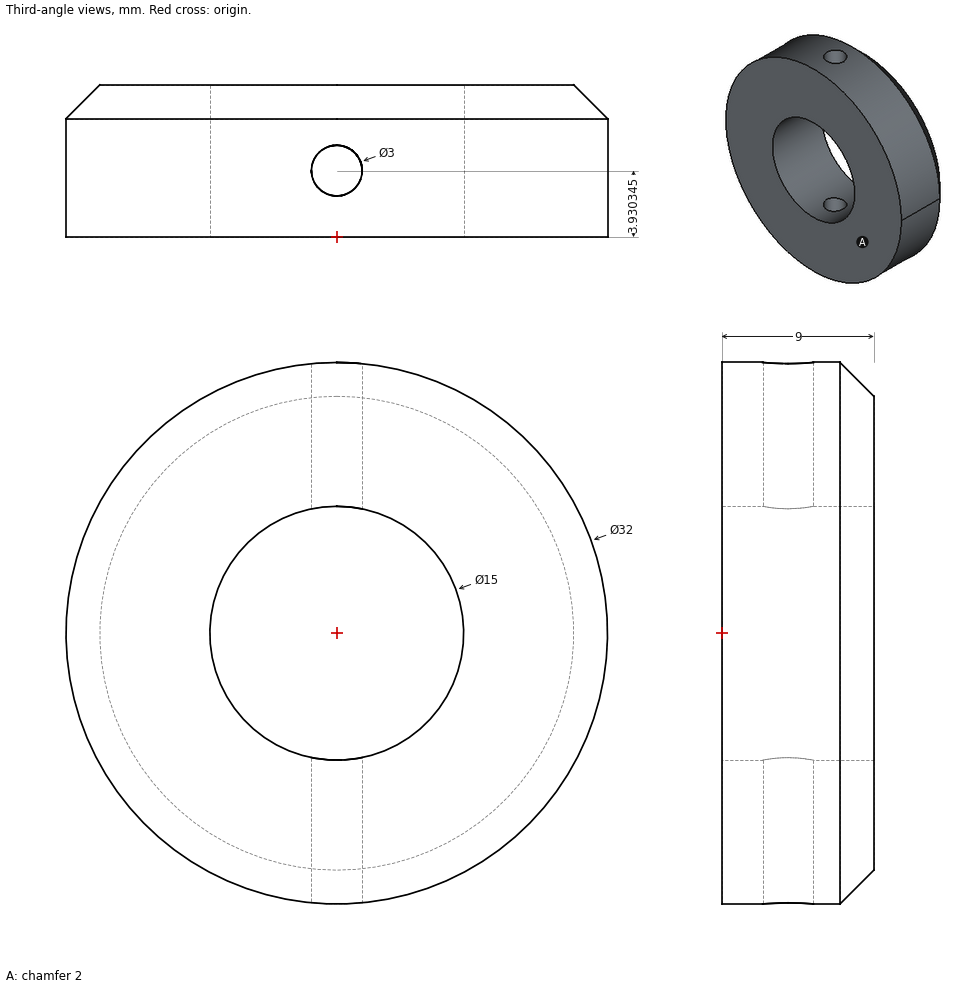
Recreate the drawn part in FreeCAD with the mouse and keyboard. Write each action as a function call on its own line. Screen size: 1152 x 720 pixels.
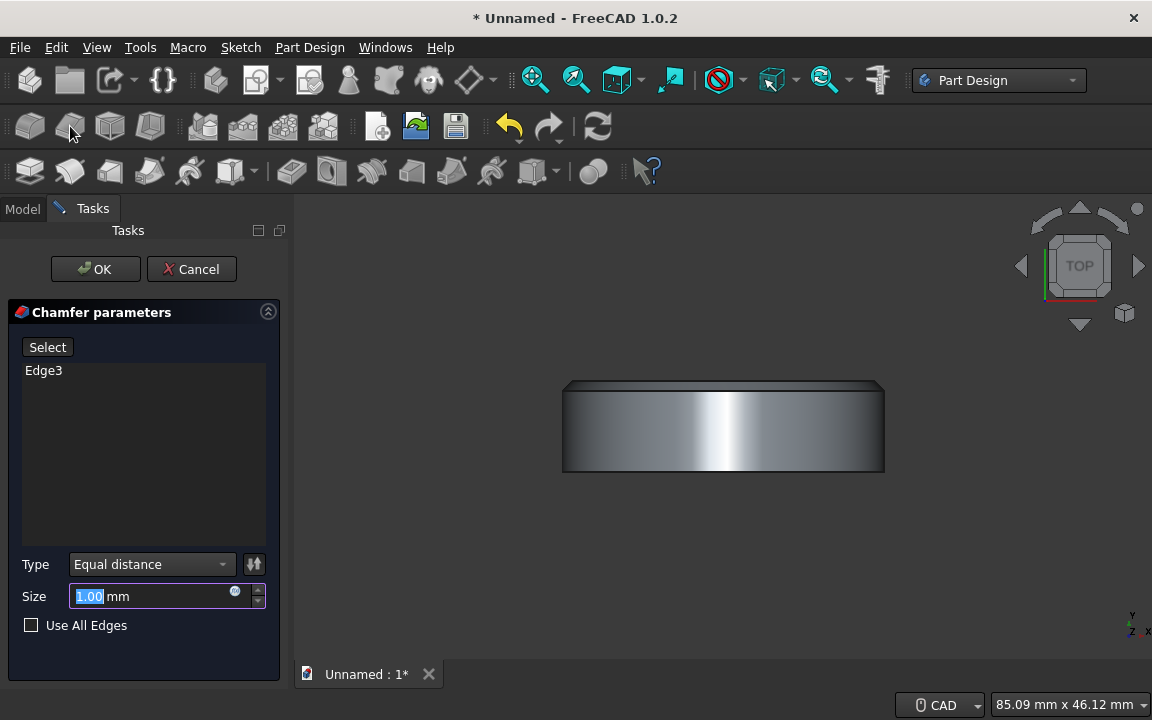
text(2)
key(Tab)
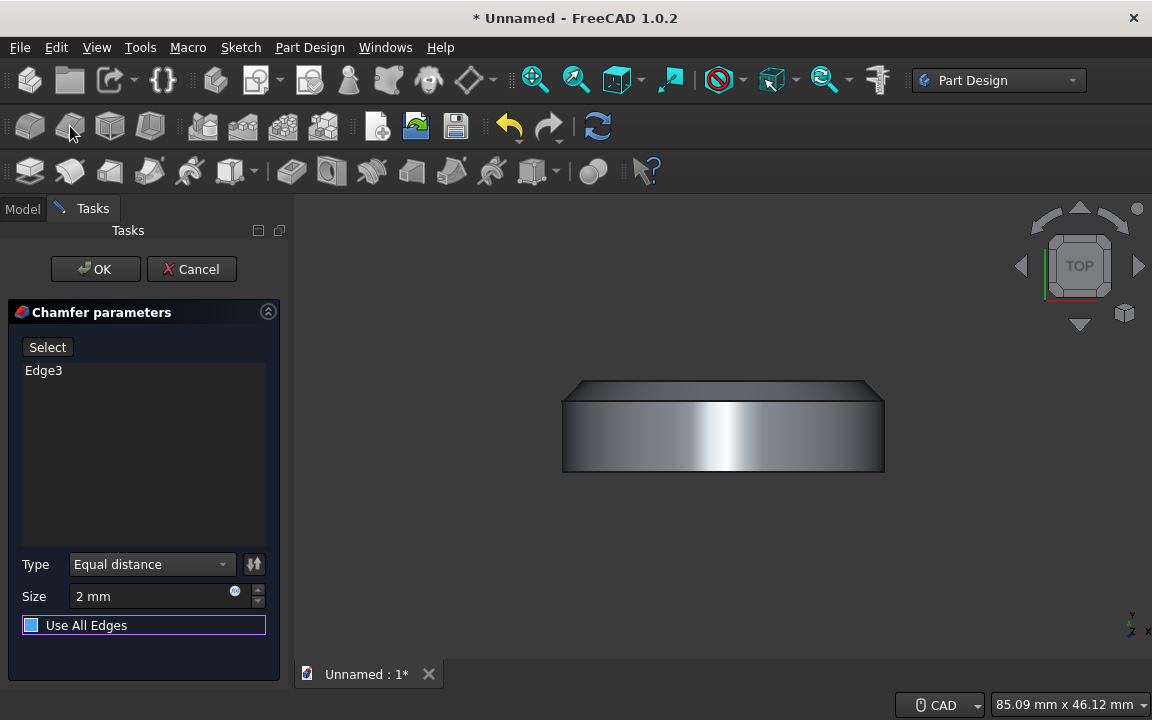
click(96, 269)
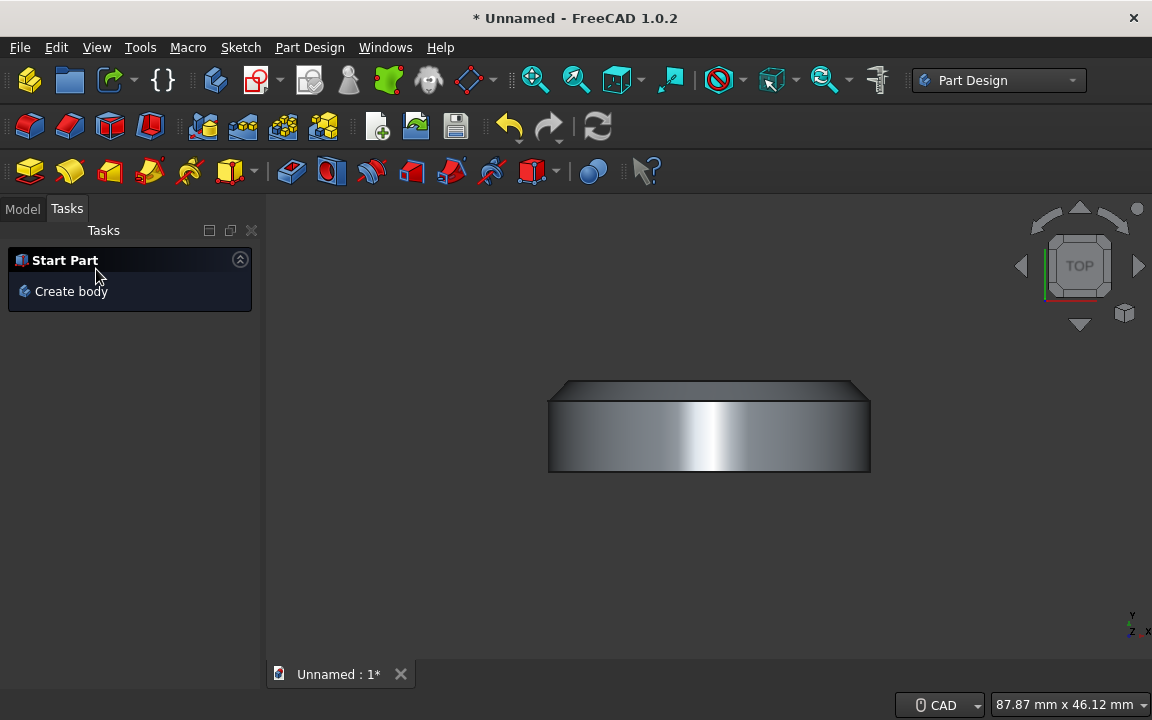
click(536, 80)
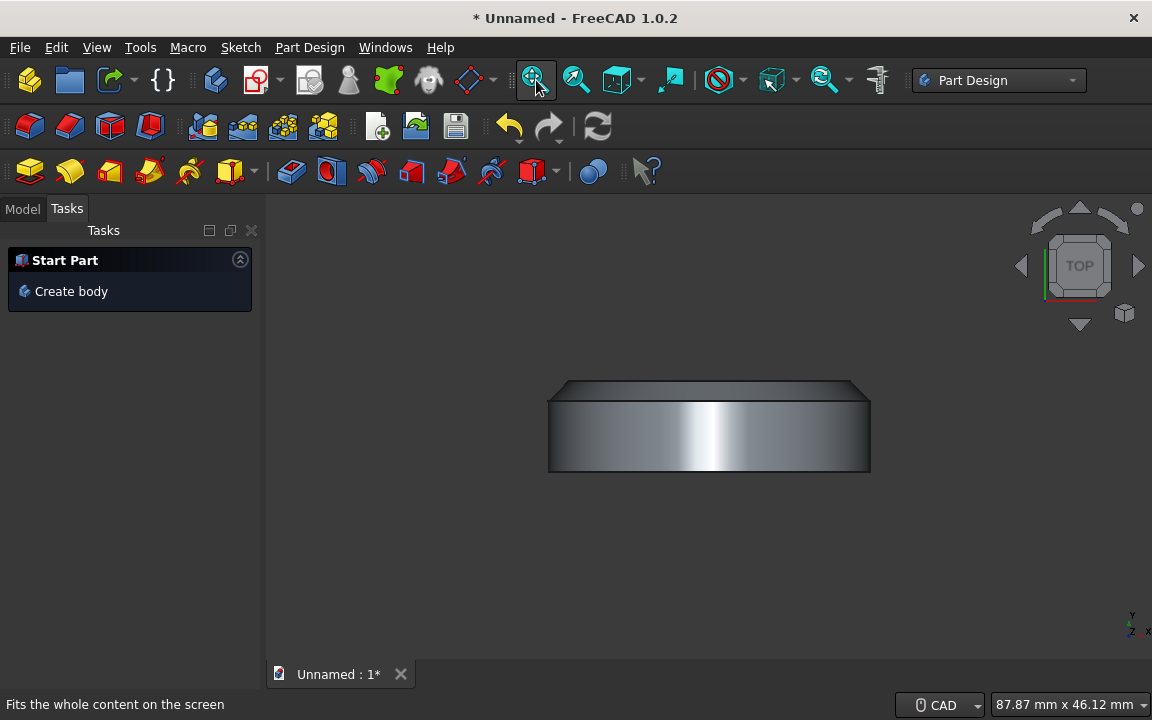
click(256, 80)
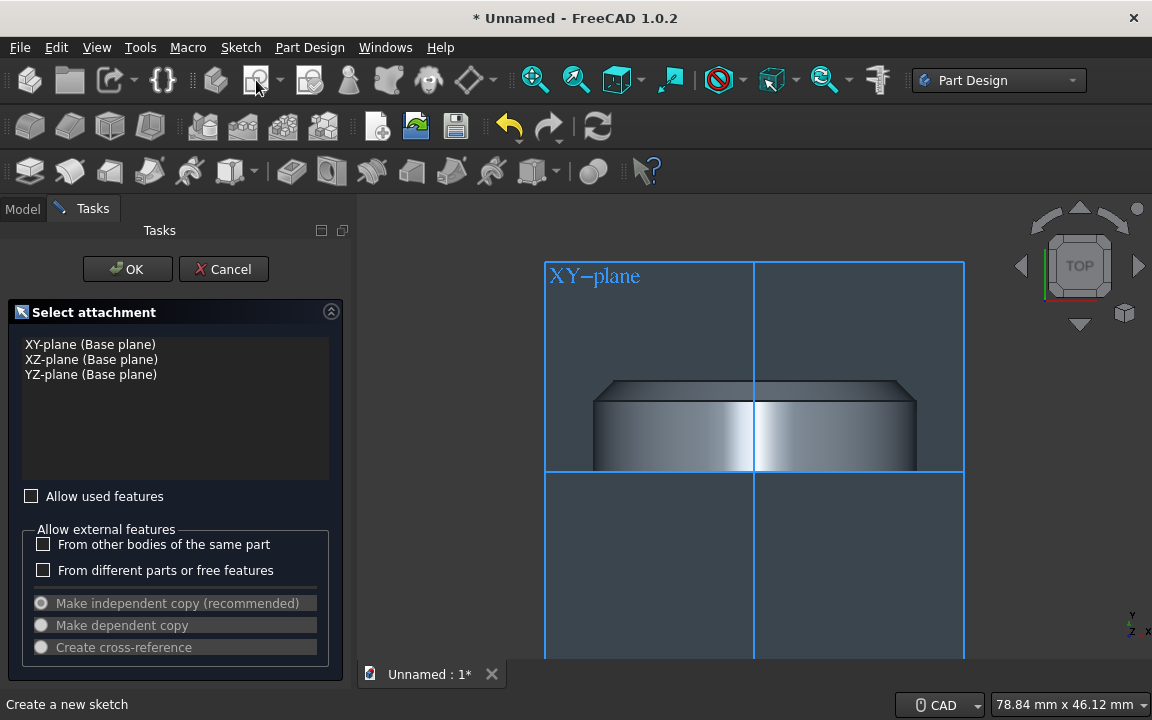
click(82, 344)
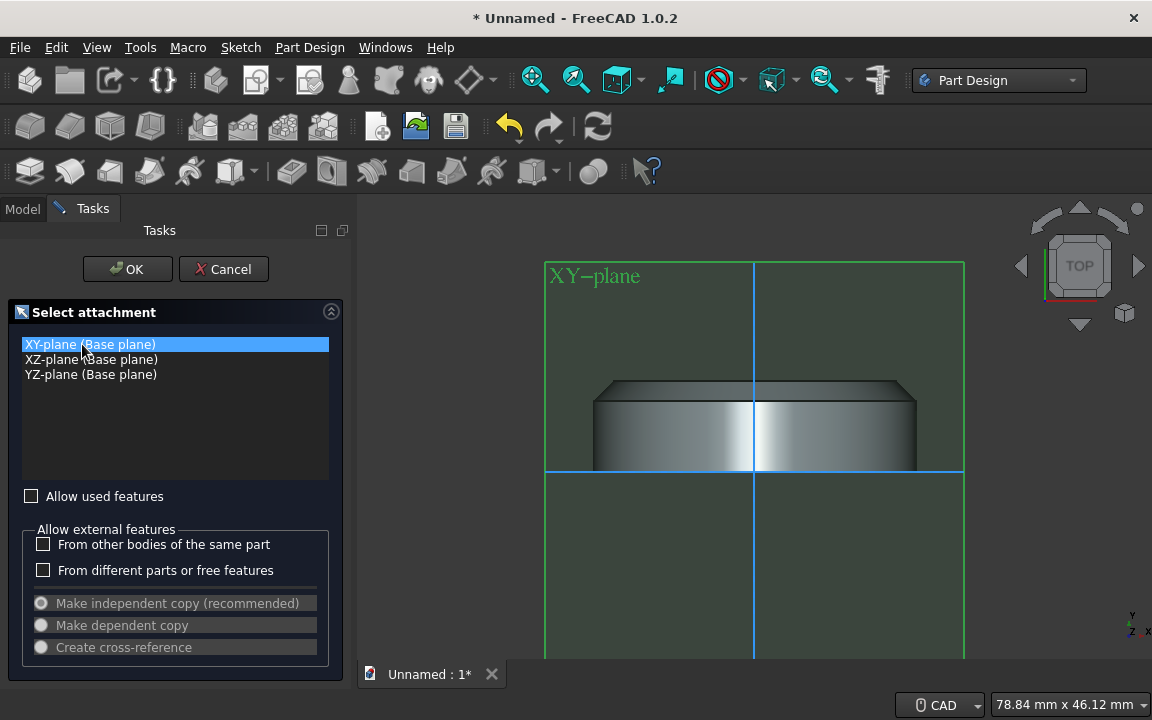
click(128, 269)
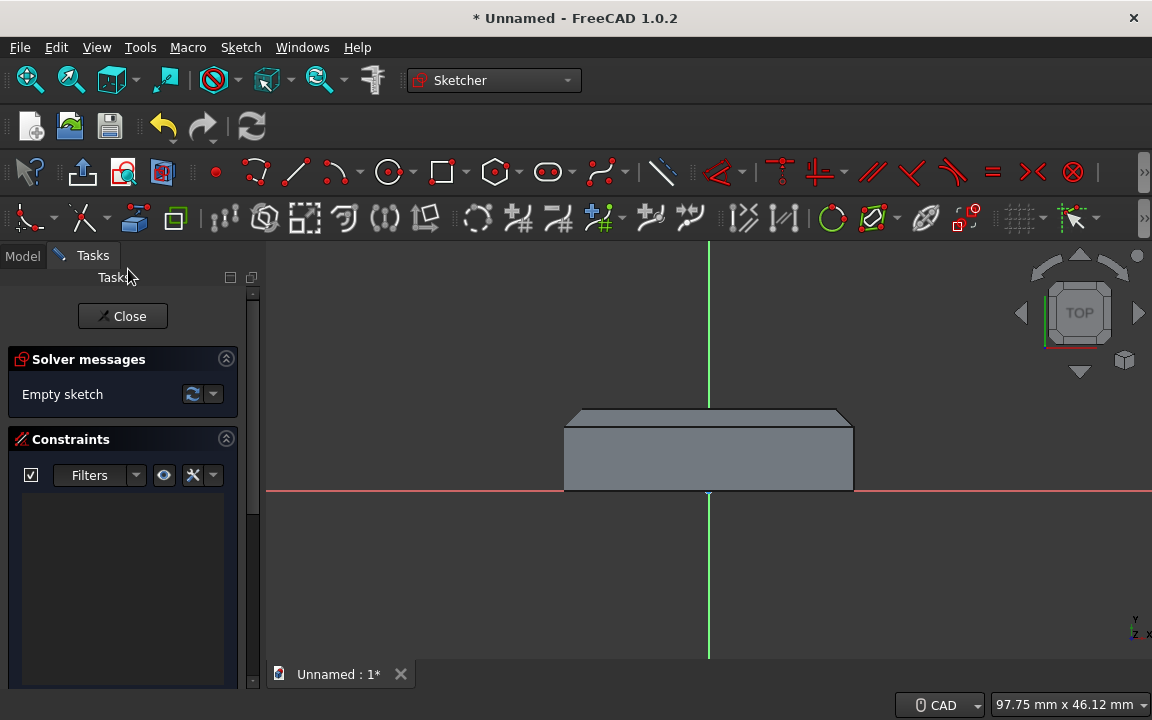
click(164, 172)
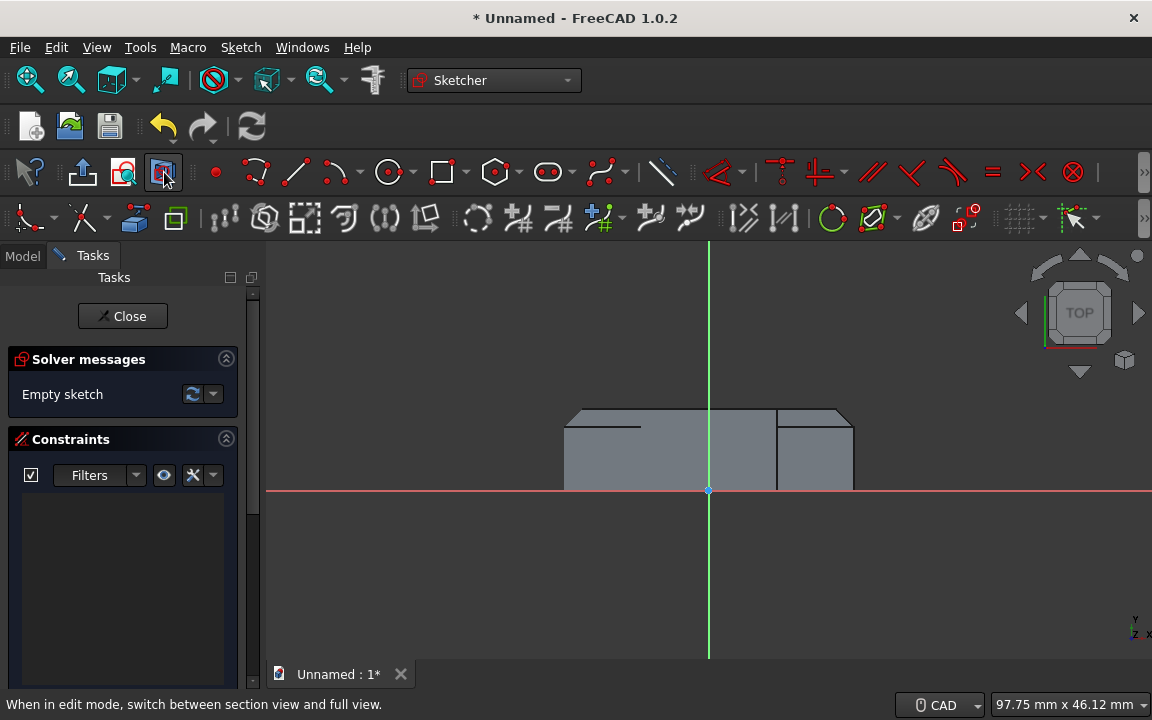
scroll(726, 470, up, 8)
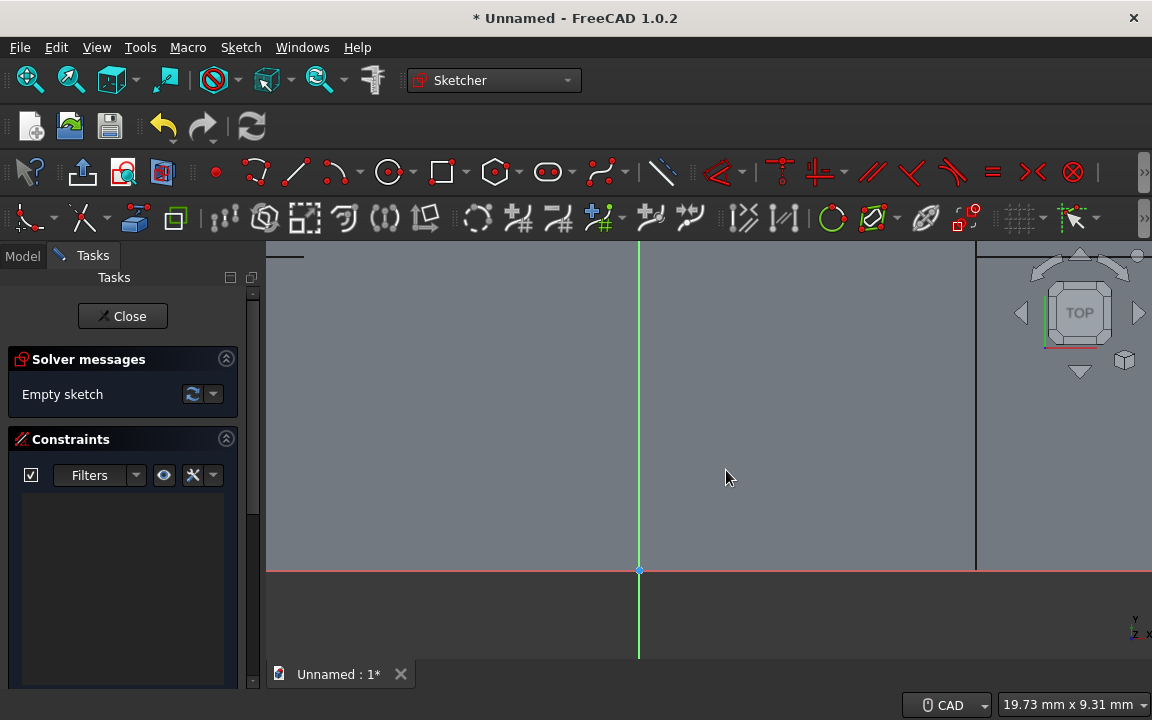
click(390, 172)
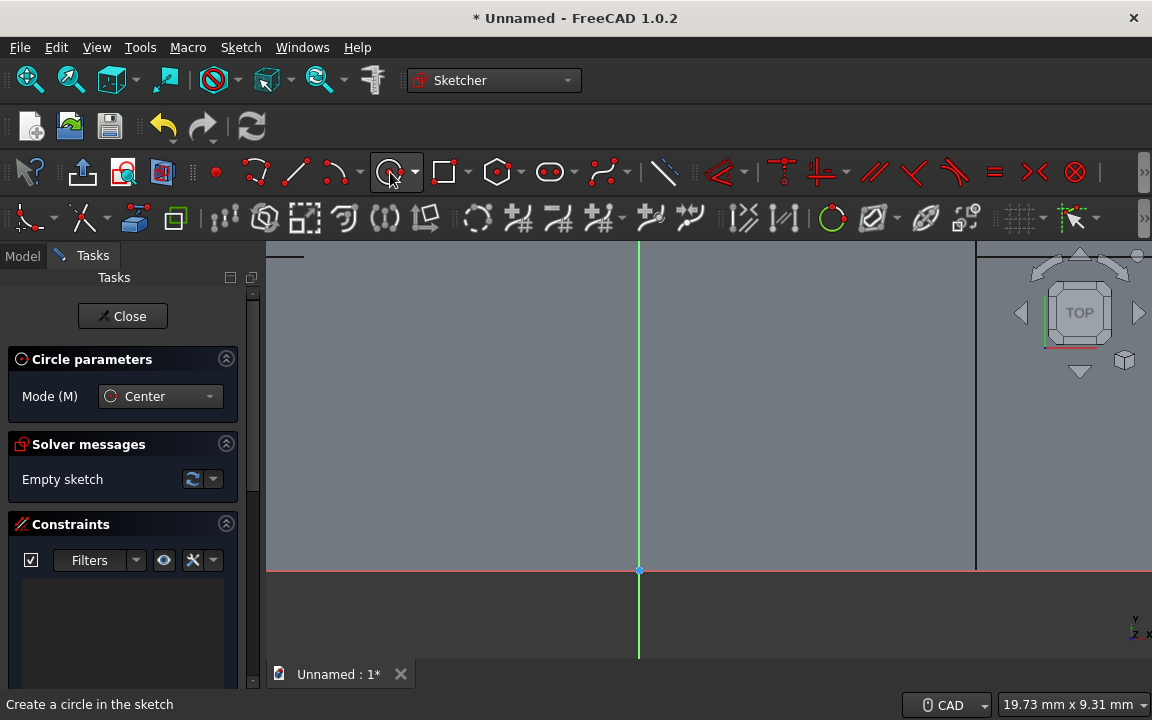
click(639, 394)
click(687, 347)
key(Escape)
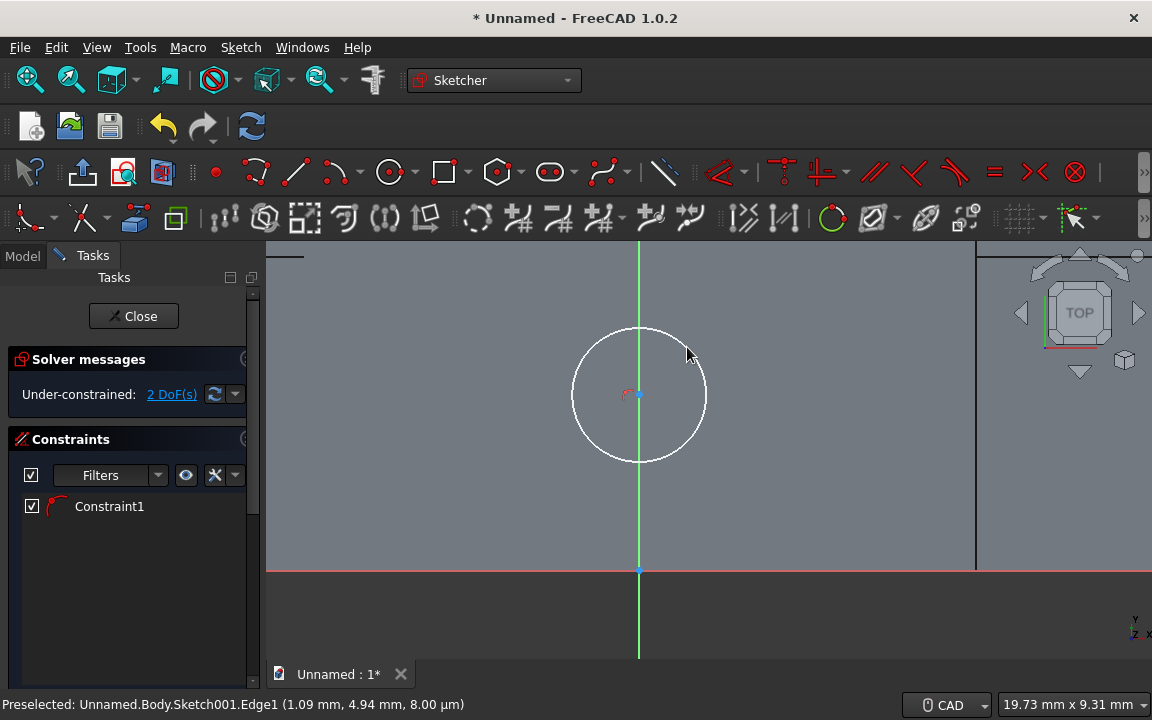
key(d)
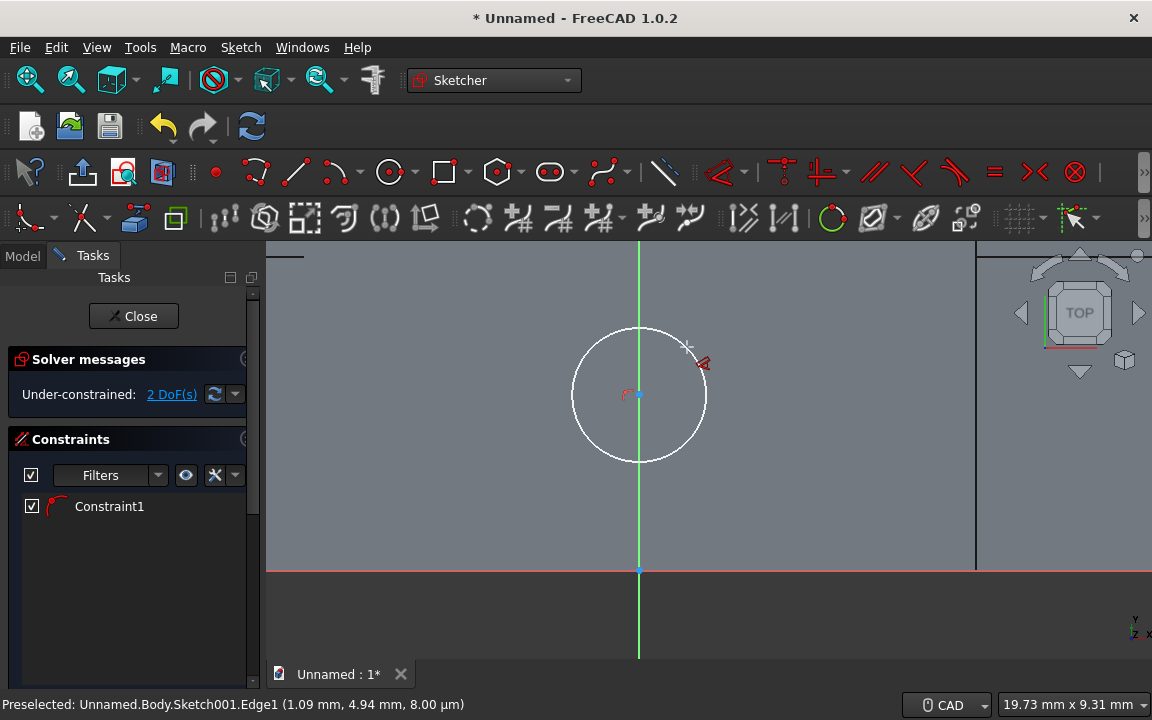
click(686, 347)
click(708, 324)